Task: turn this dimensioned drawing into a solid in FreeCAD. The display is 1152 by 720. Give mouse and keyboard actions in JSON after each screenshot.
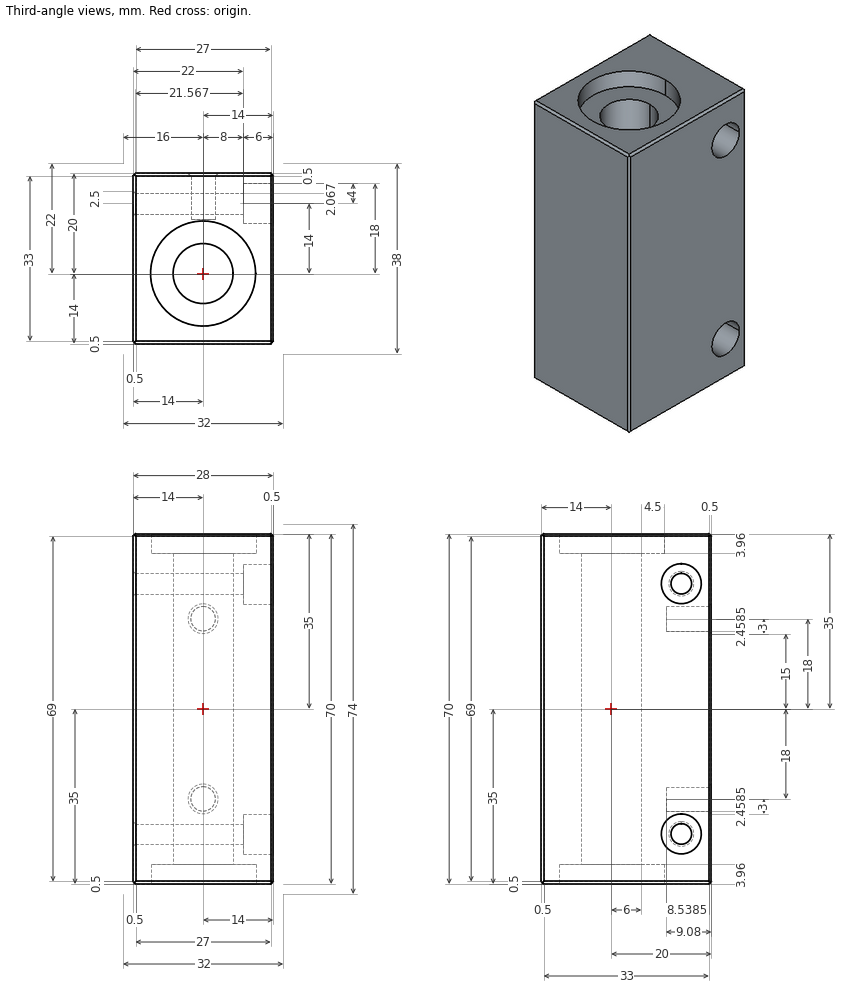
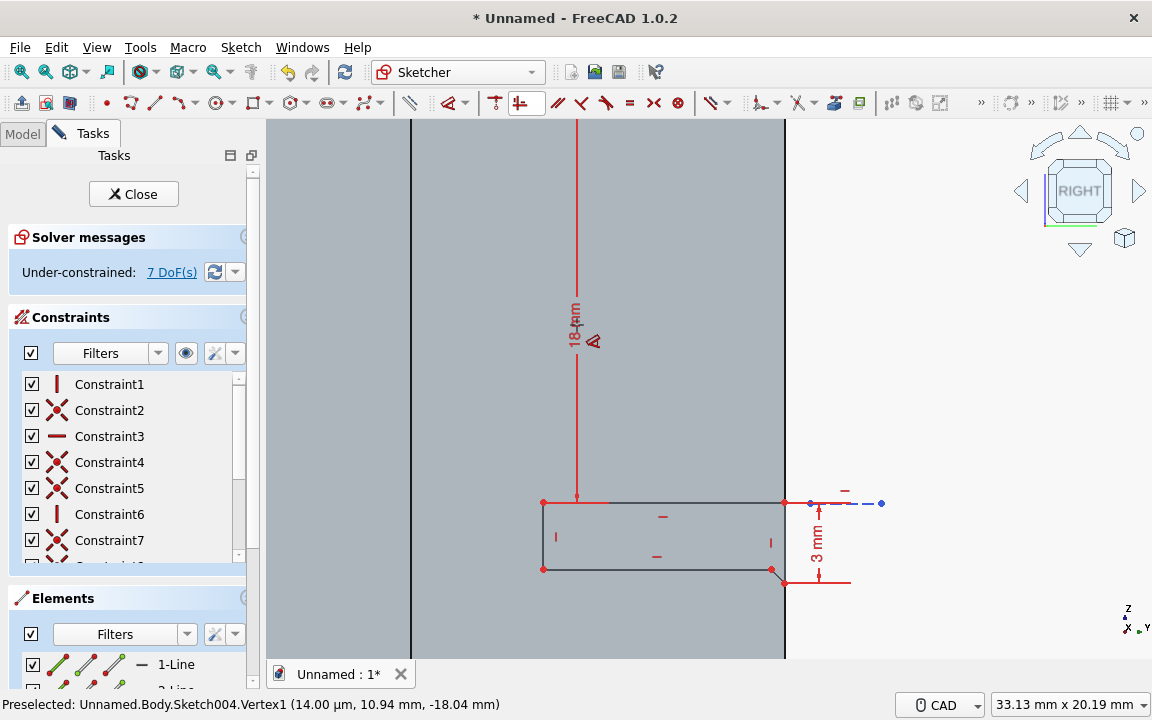
{"action": "left_click", "coordinate": [785, 583]}
{"action": "left_click", "coordinate": [539, 617]}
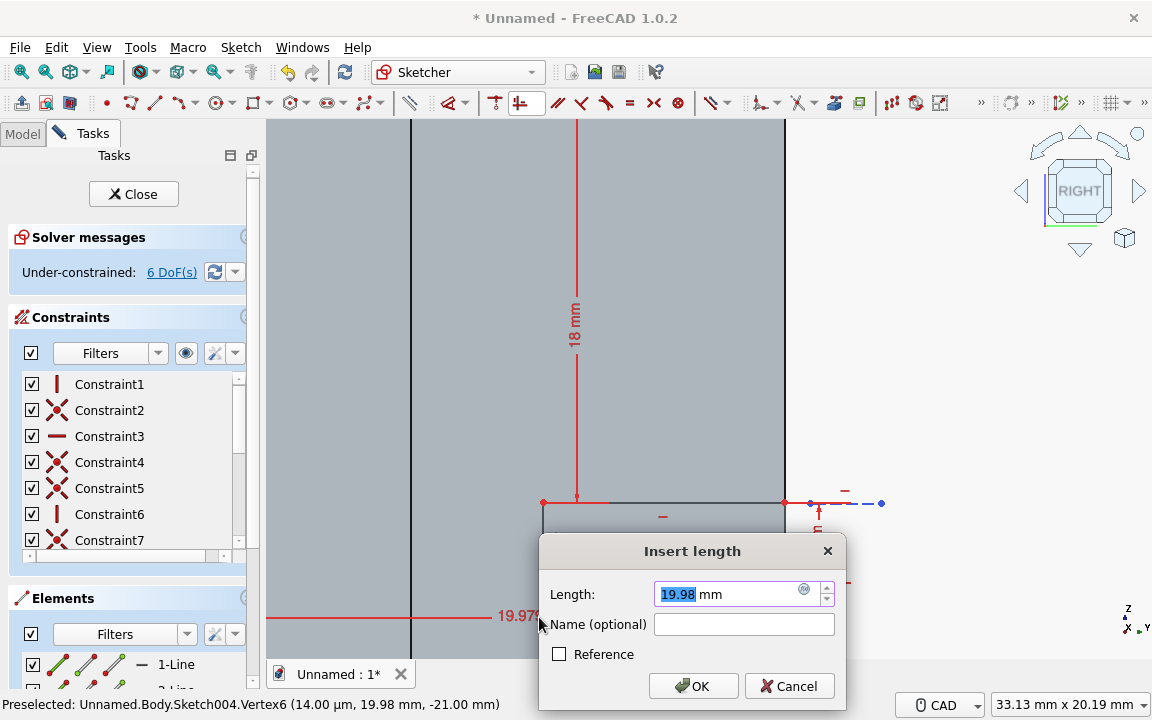
{"action": "type", "text": "20"}
{"action": "key", "text": "Return"}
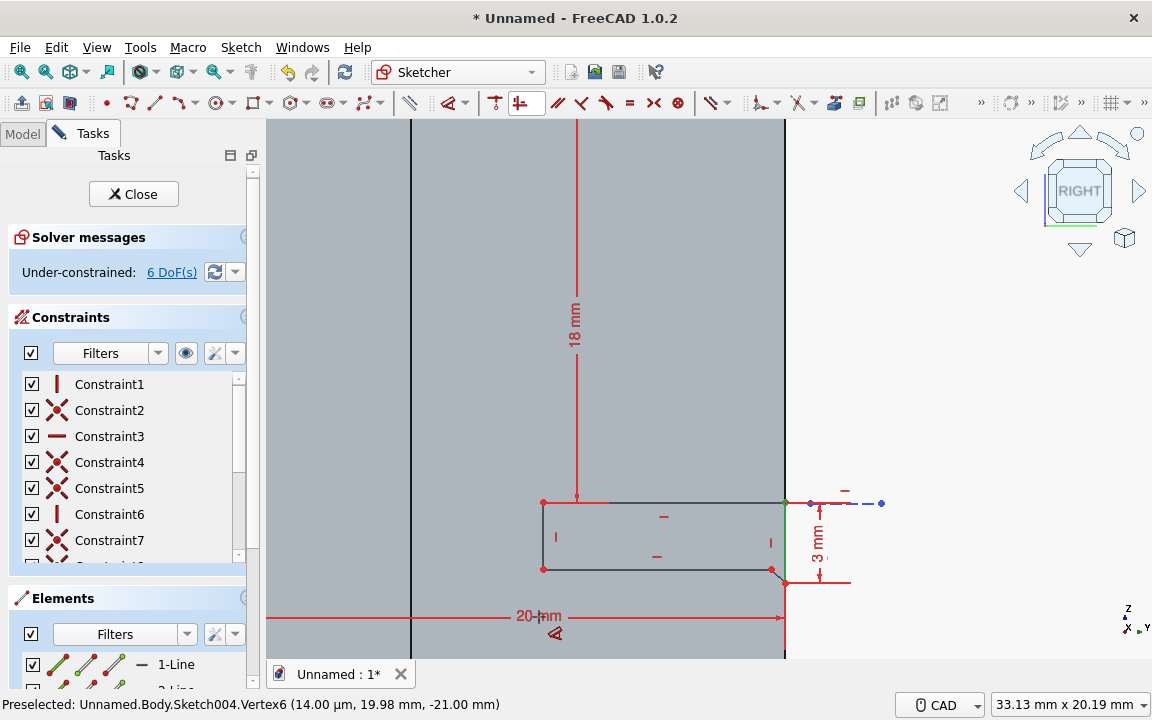
{"action": "left_click", "coordinate": [810, 504]}
{"action": "left_click", "coordinate": [844, 325]}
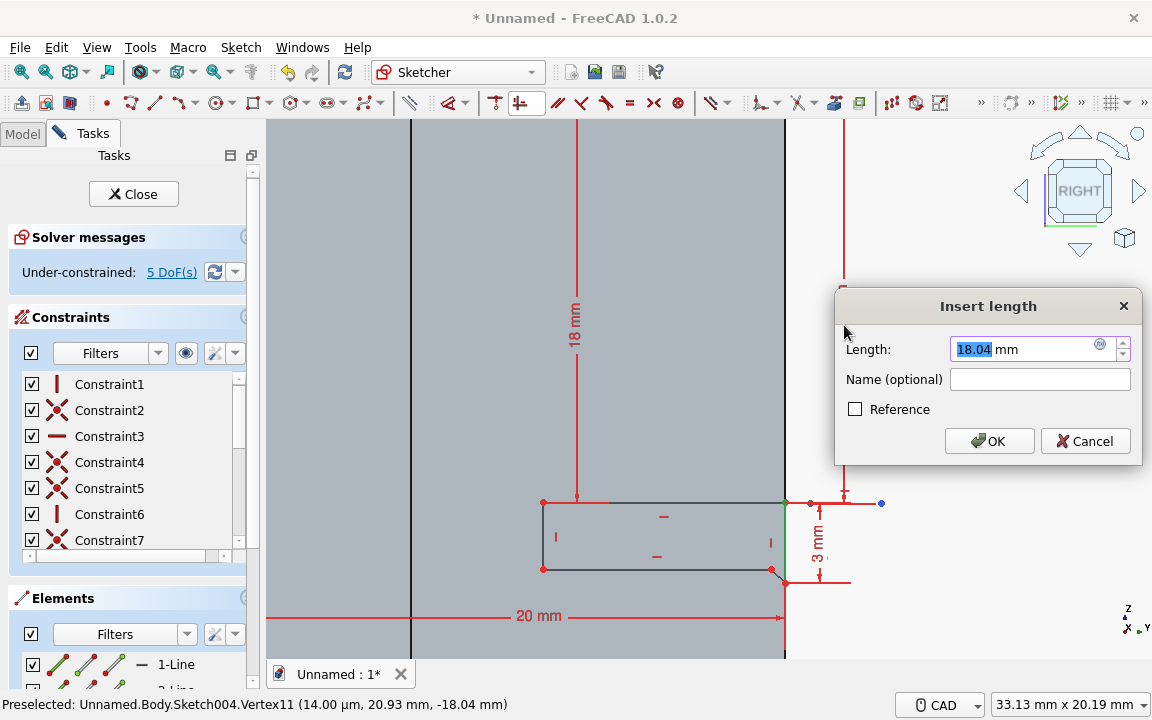
{"action": "type", "text": "18"}
{"action": "key", "text": "Return"}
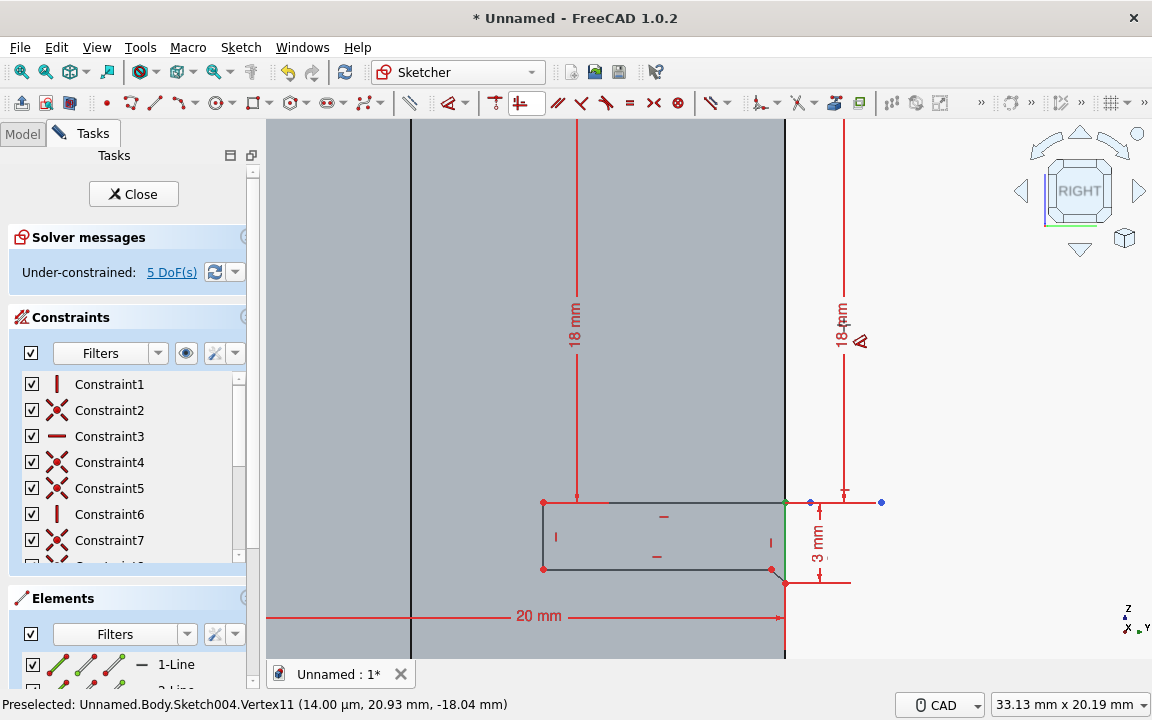
{"action": "left_click", "coordinate": [713, 503]}
{"action": "left_click", "coordinate": [664, 537]}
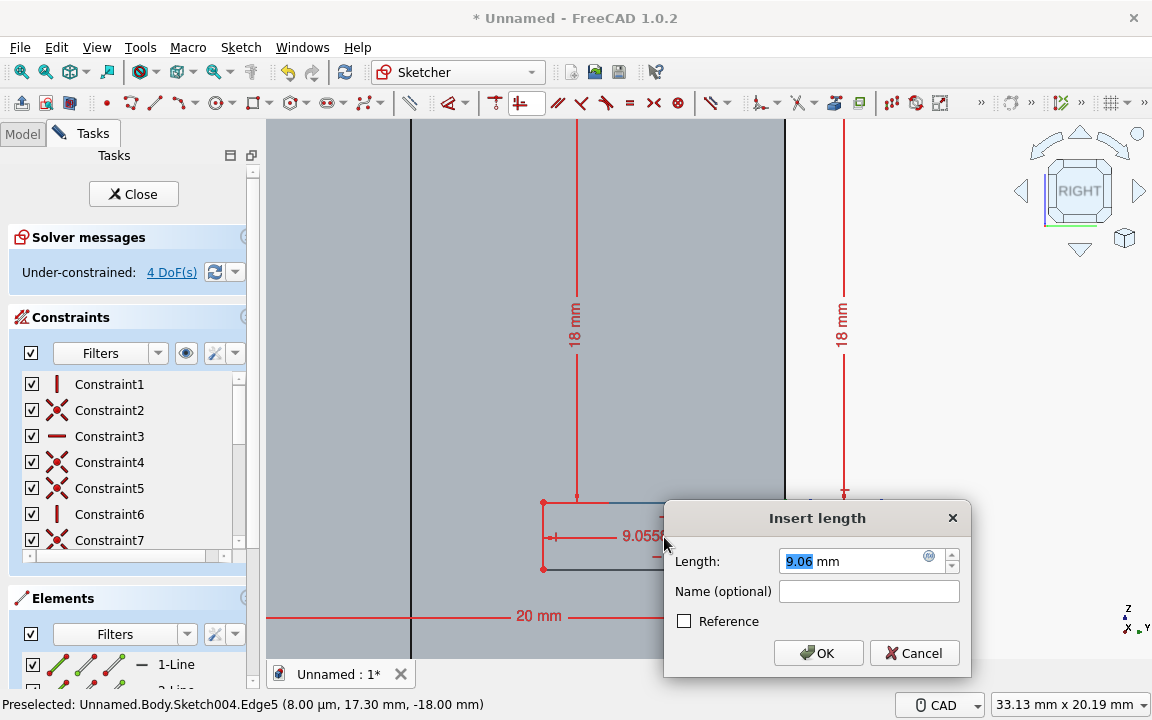
{"action": "type", "text": "9.08"}
{"action": "key", "text": "Return"}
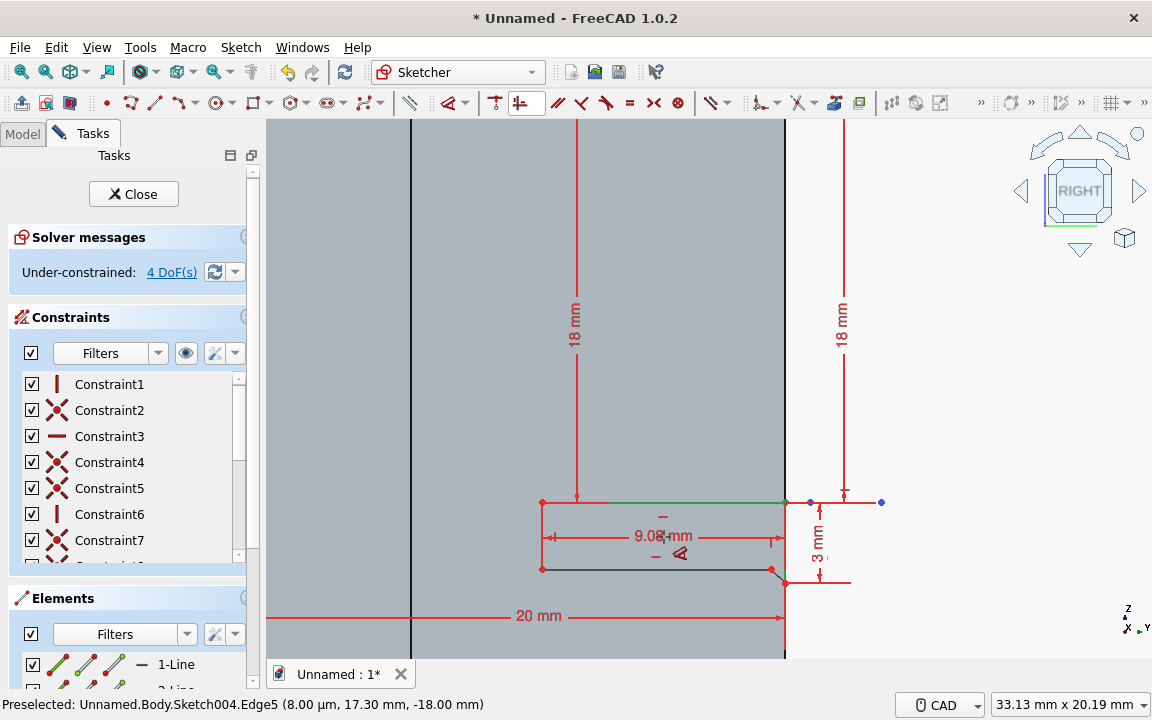
{"action": "left_click", "coordinate": [542, 523]}
{"action": "left_click", "coordinate": [508, 536]}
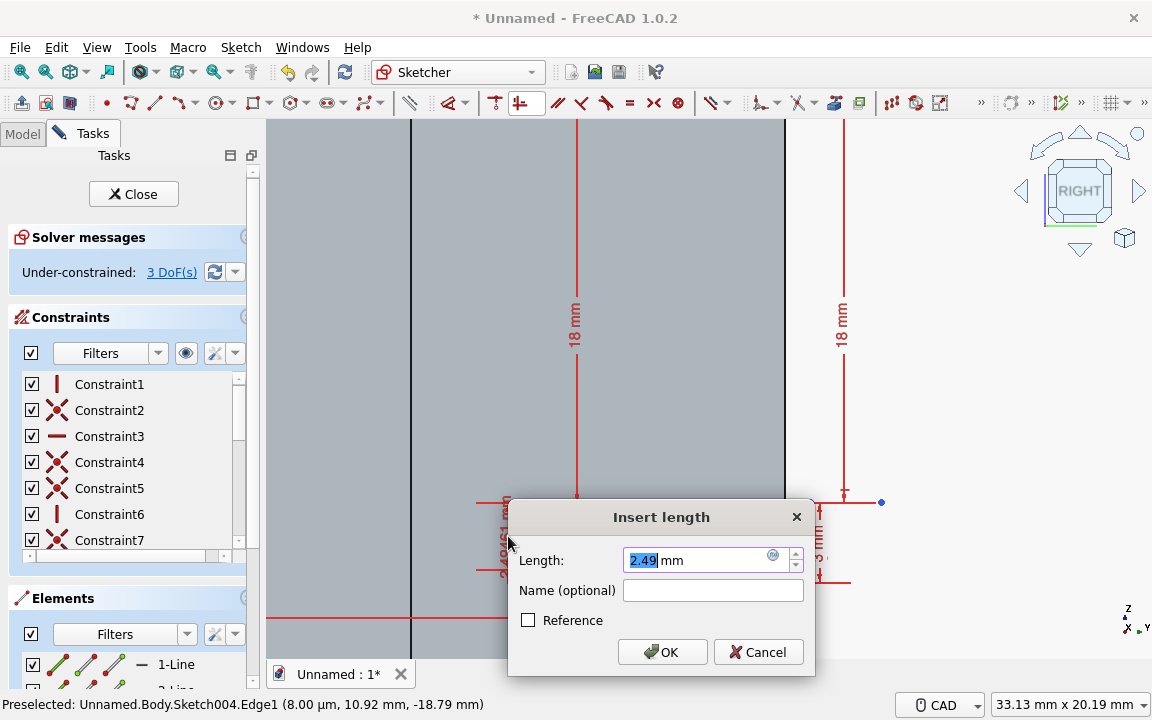
{"action": "type", "text": "2.4585"}
{"action": "key", "text": "Return"}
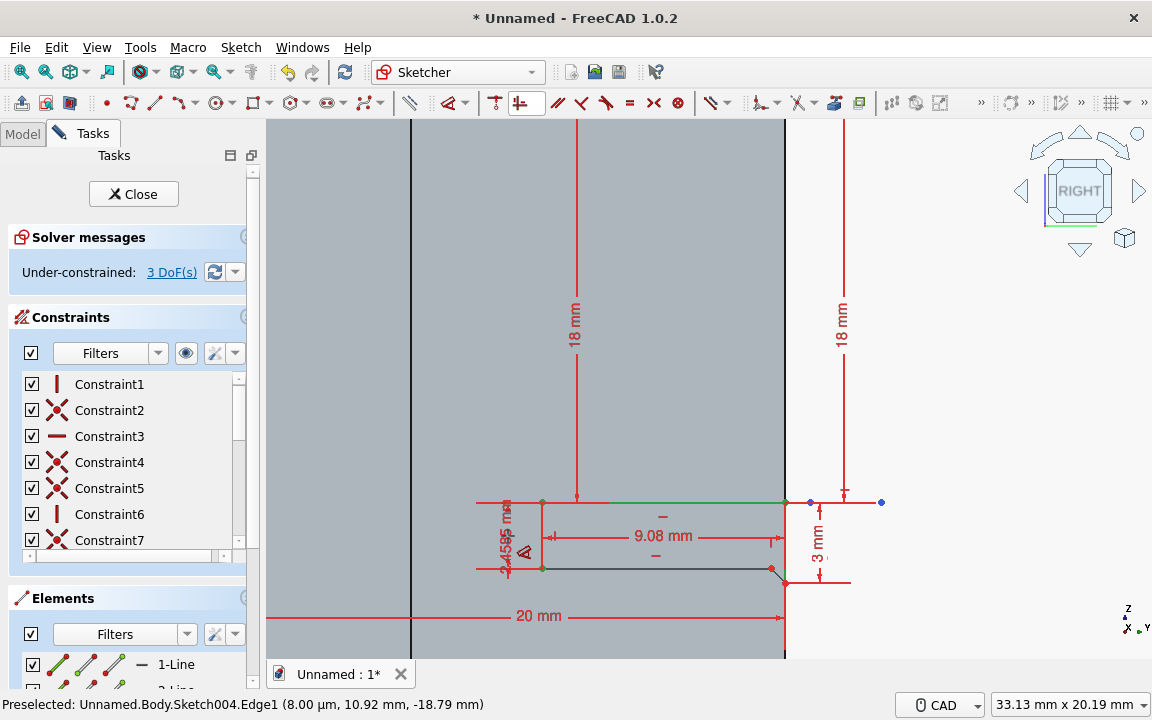
{"action": "left_click", "coordinate": [611, 569]}
{"action": "left_click", "coordinate": [657, 603]}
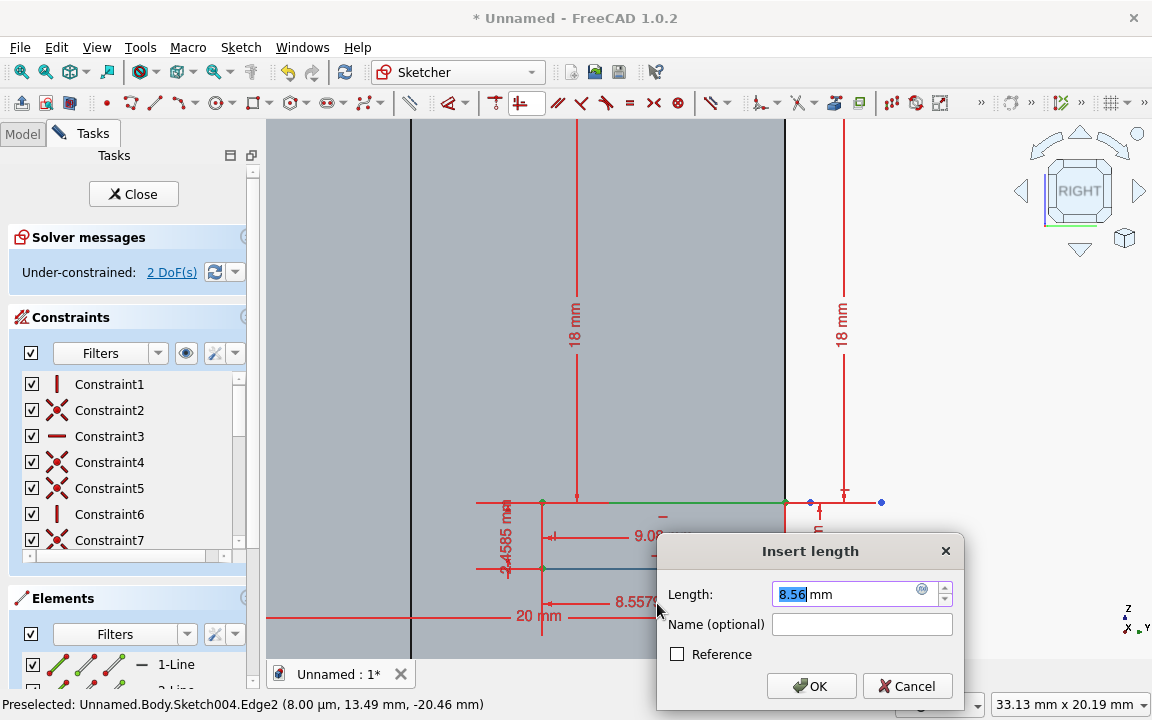
{"action": "type", "text": "8.5385"}
{"action": "key", "text": "Return"}
{"action": "key", "text": "Escape"}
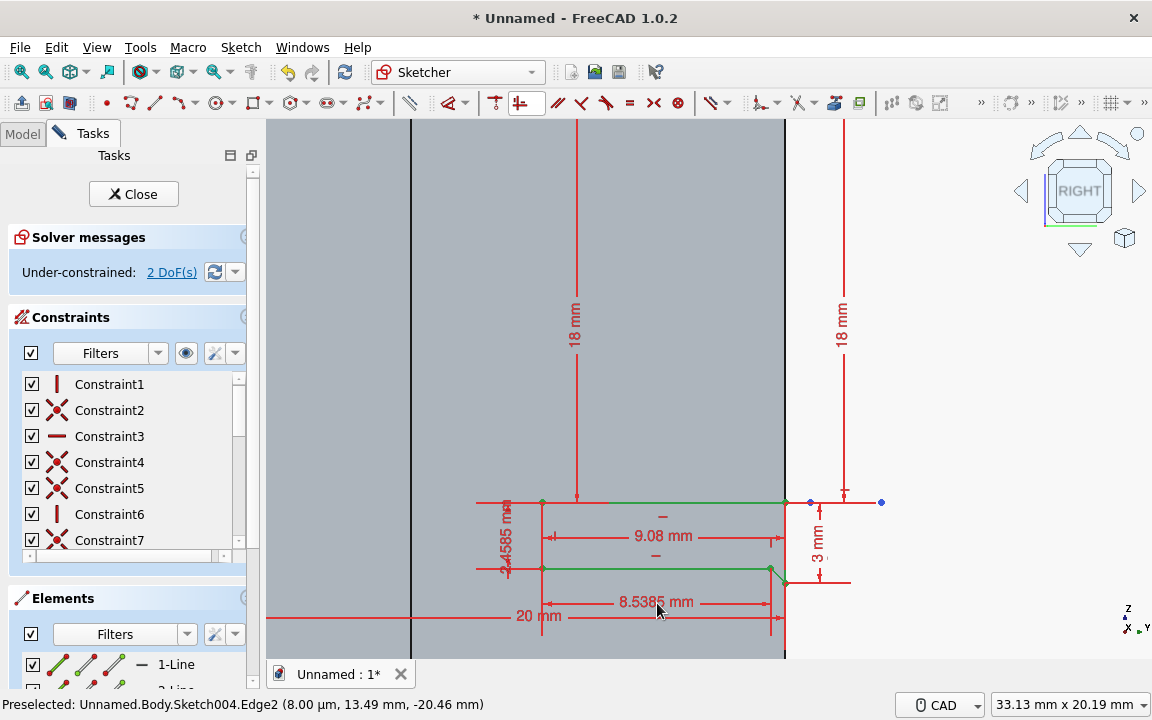
{"action": "left_click", "coordinate": [134, 194]}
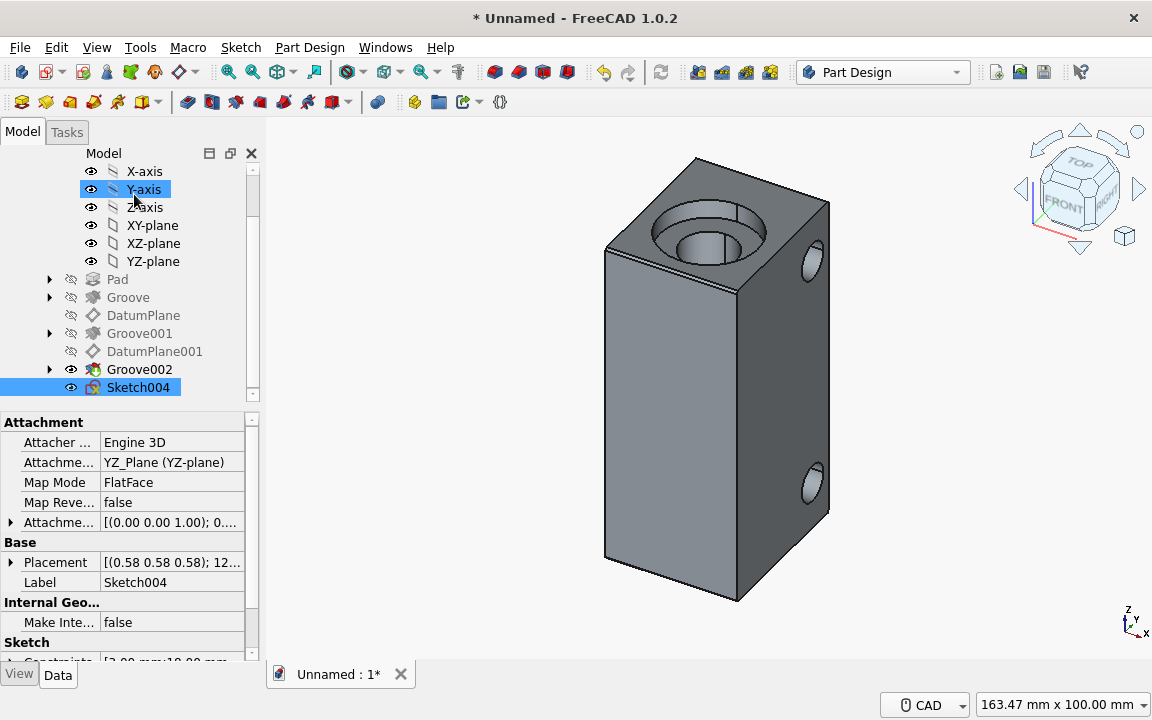
{"action": "left_click", "coordinate": [236, 102]}